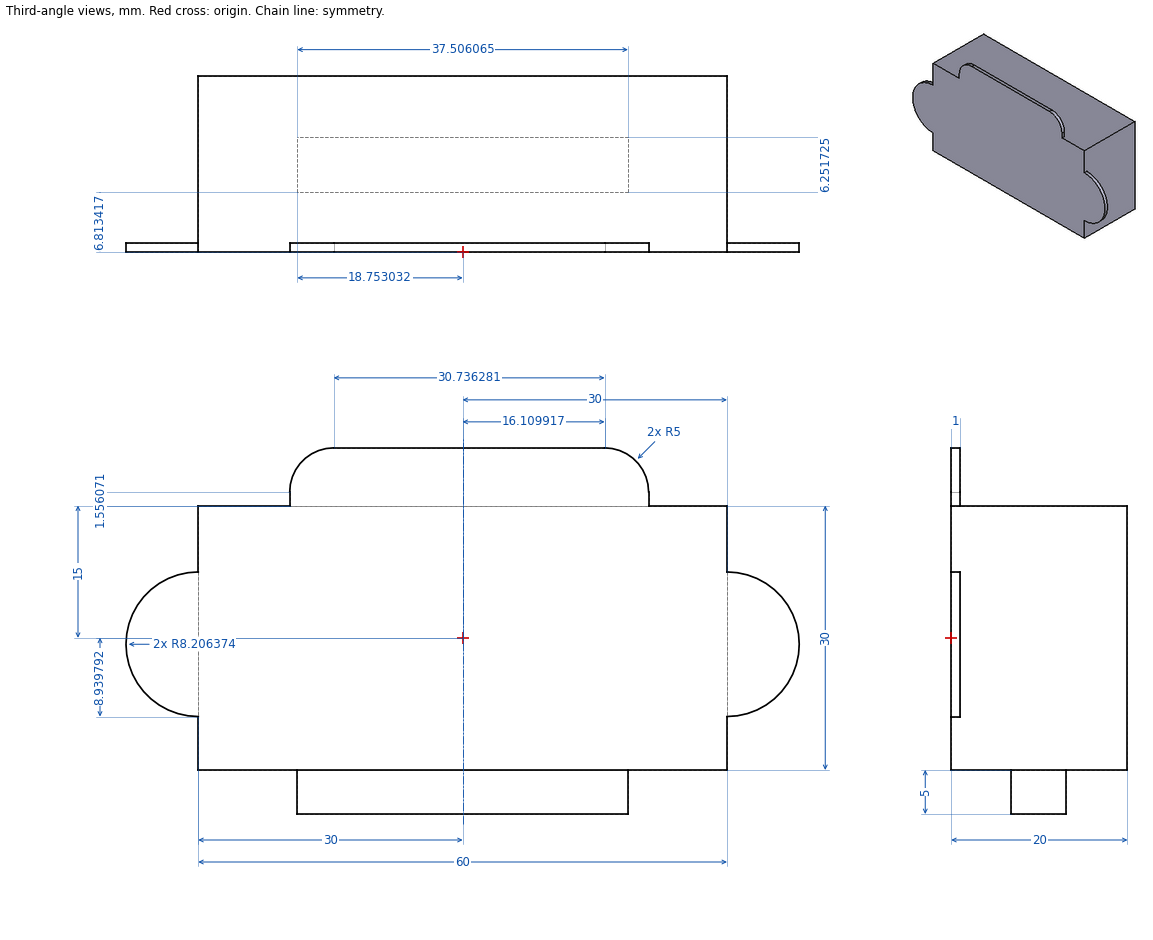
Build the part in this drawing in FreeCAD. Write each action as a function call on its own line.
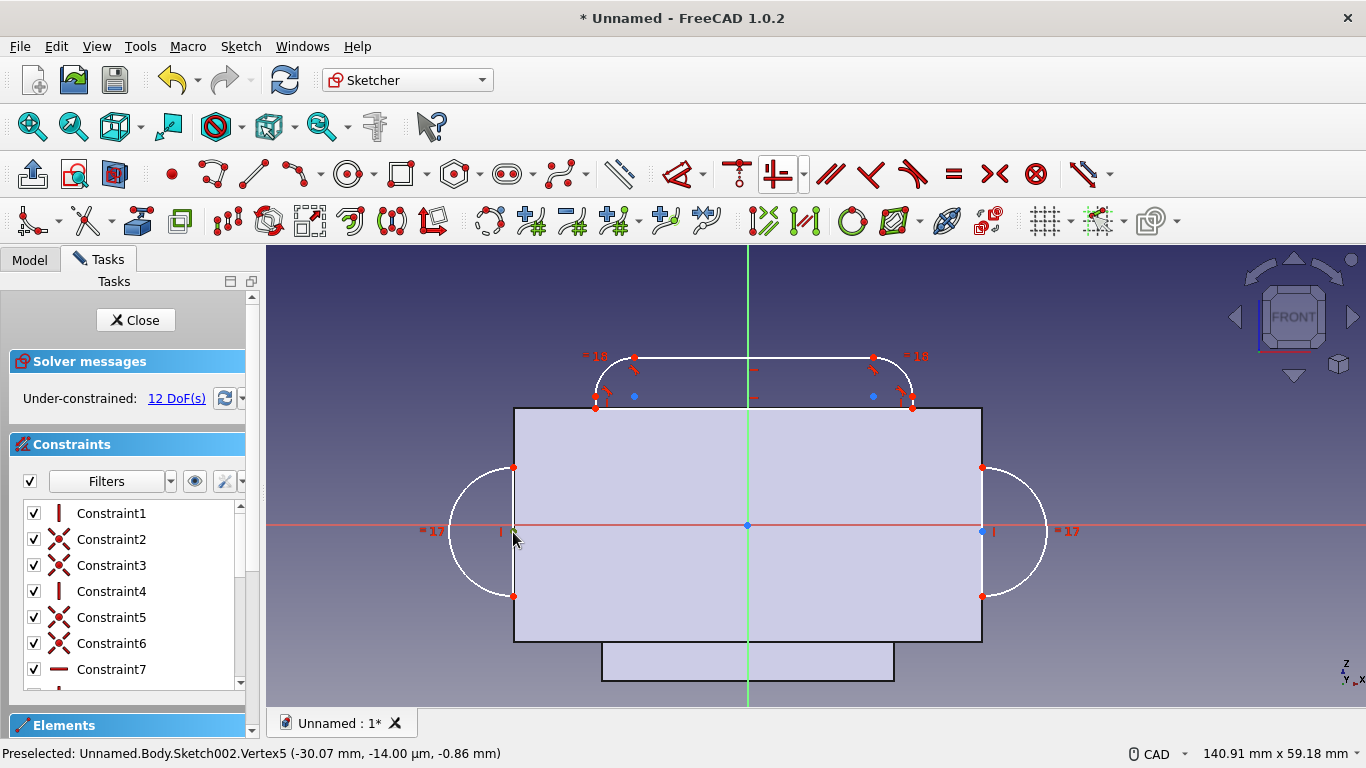
click(983, 532)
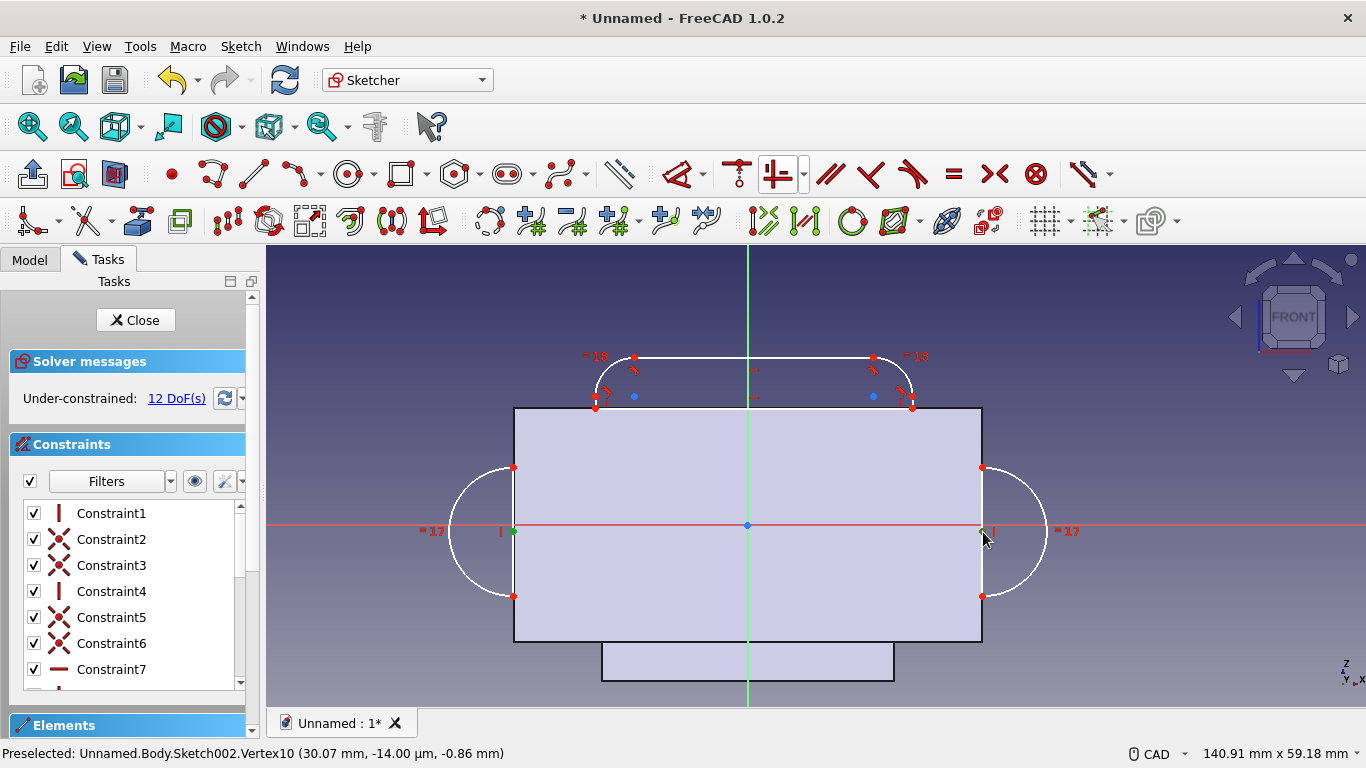
click(748, 650)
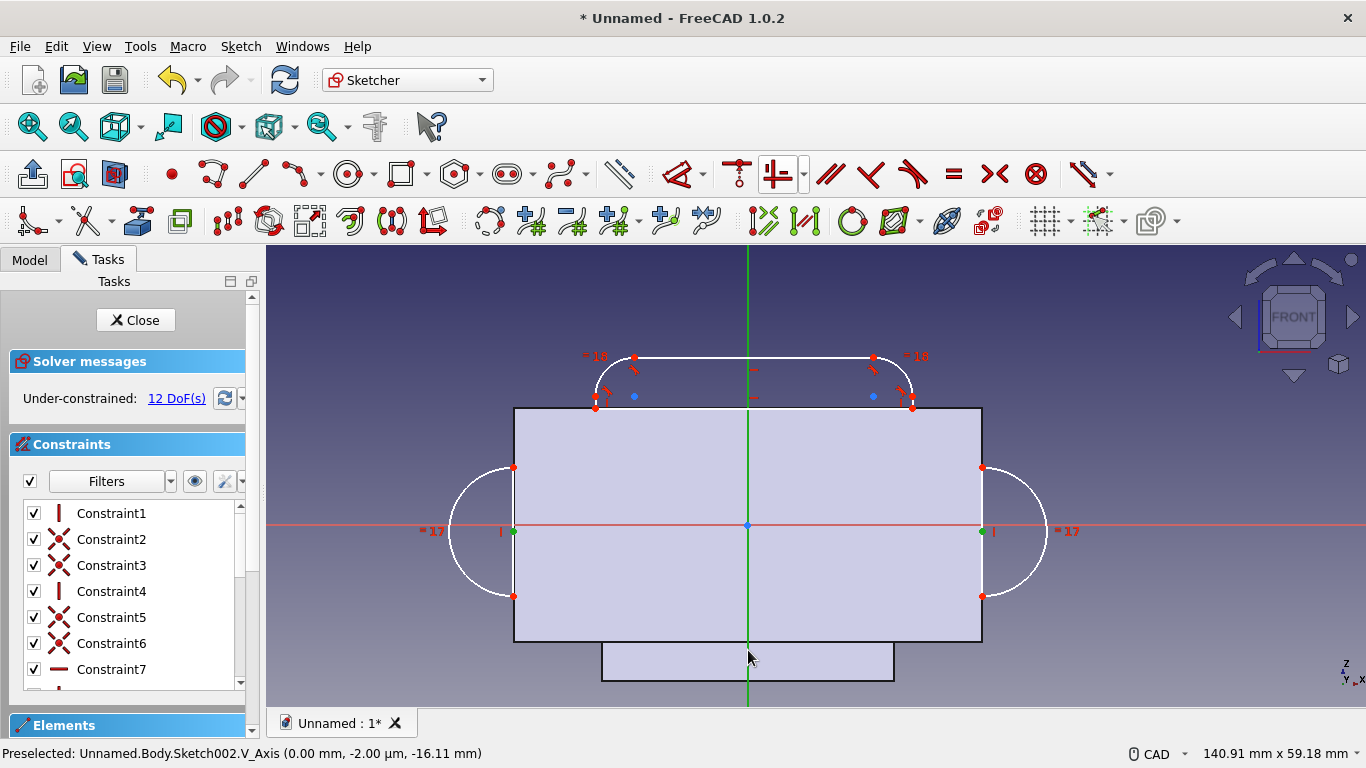
key(s)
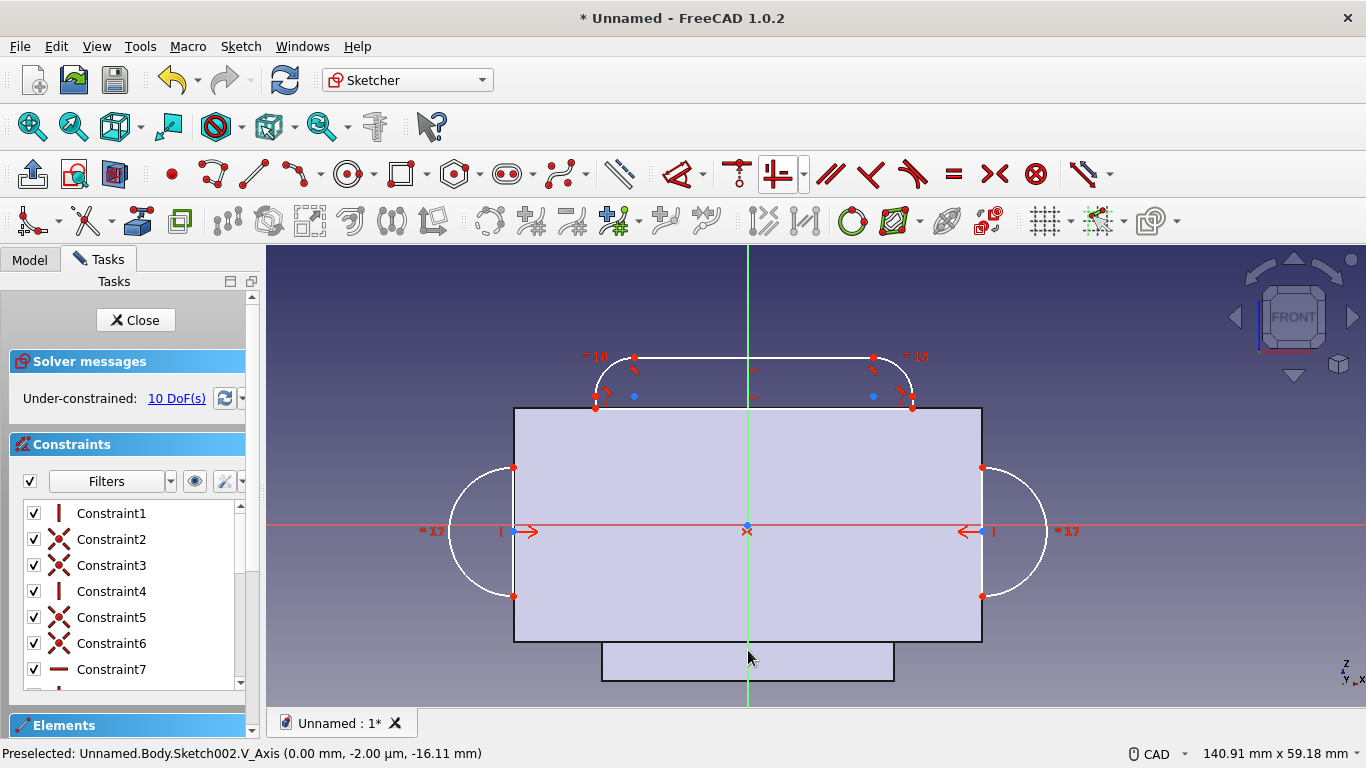
key(d)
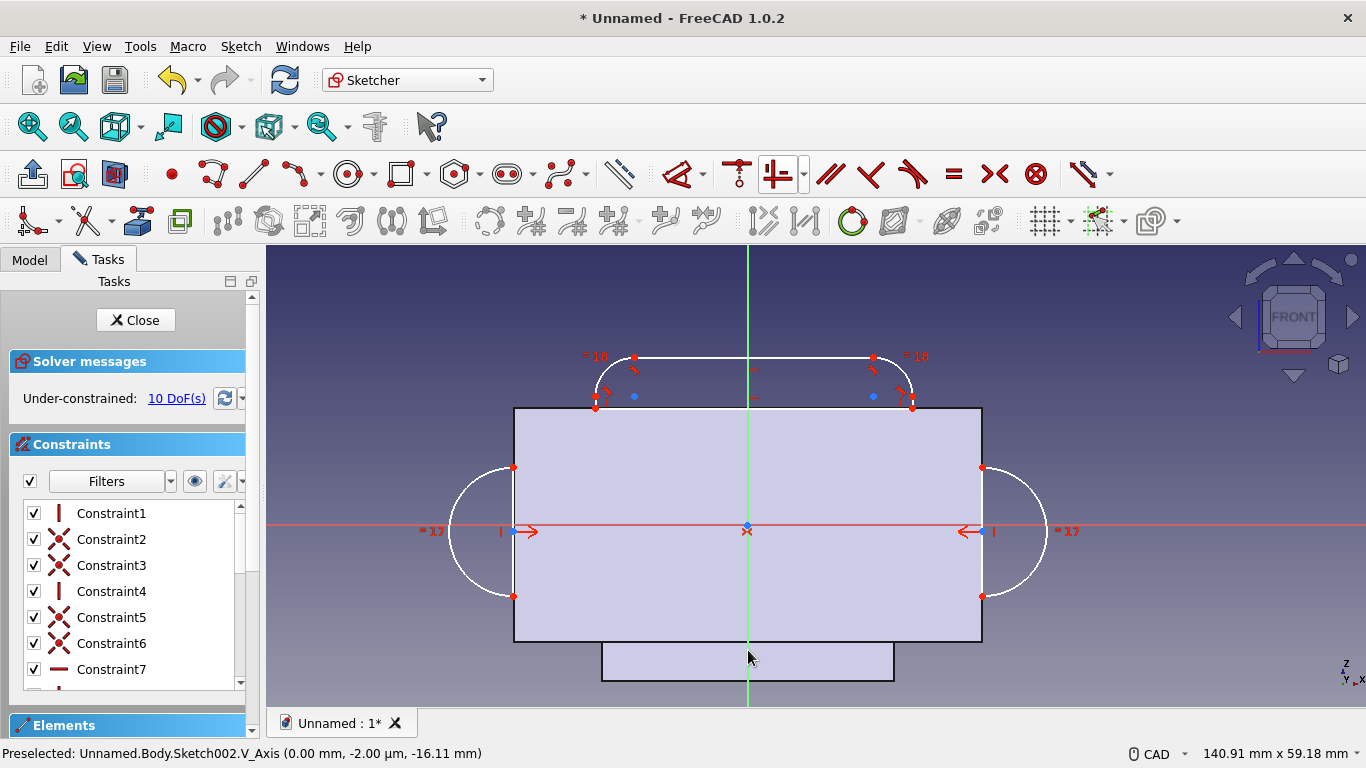
click(461, 494)
click(435, 475)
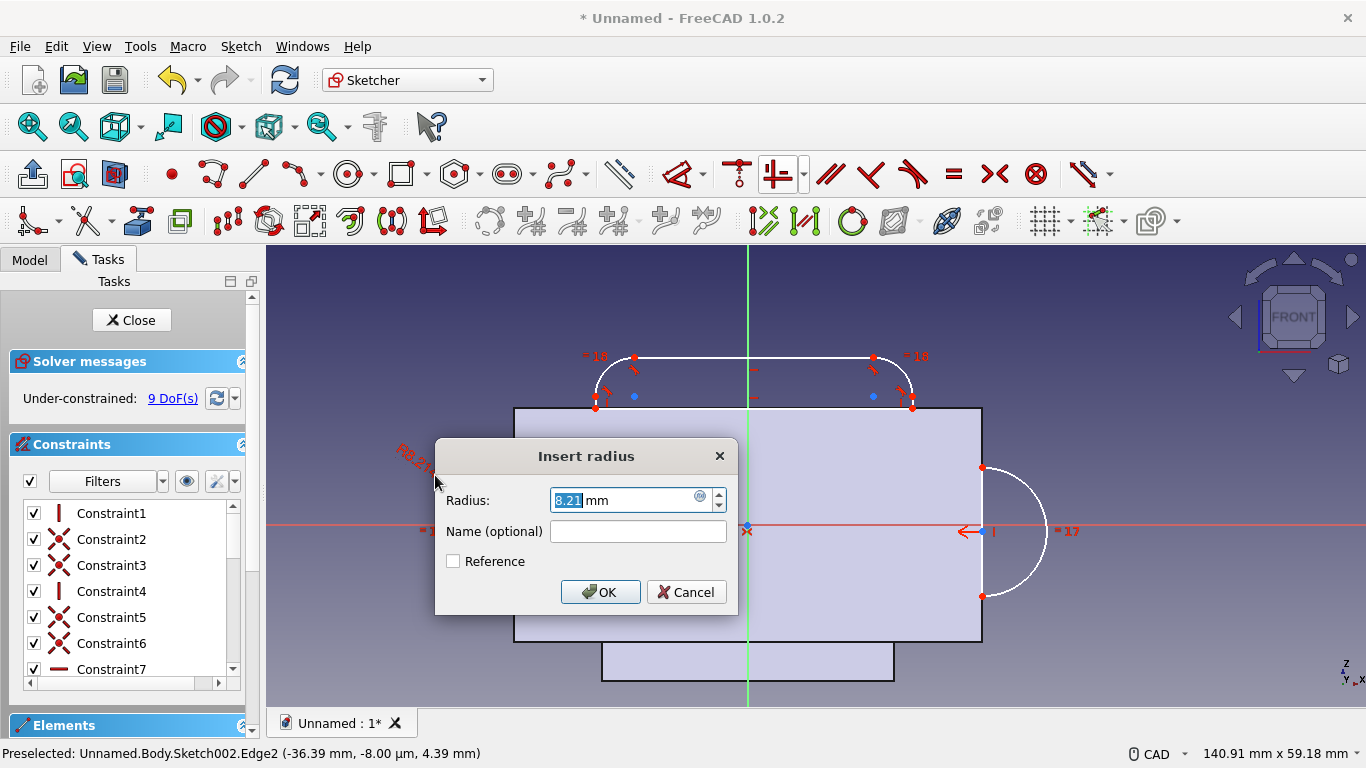
text(8.206374)
key(Return)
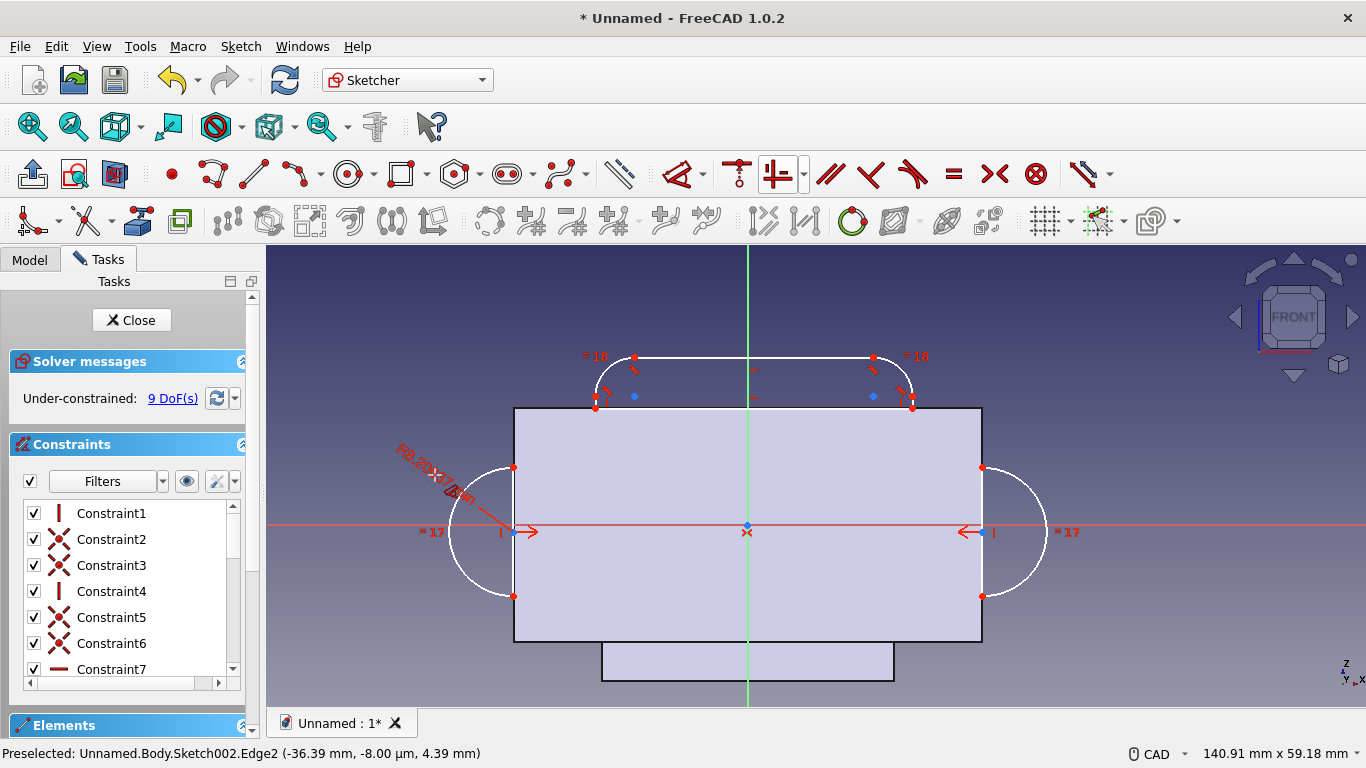
click(617, 362)
click(603, 333)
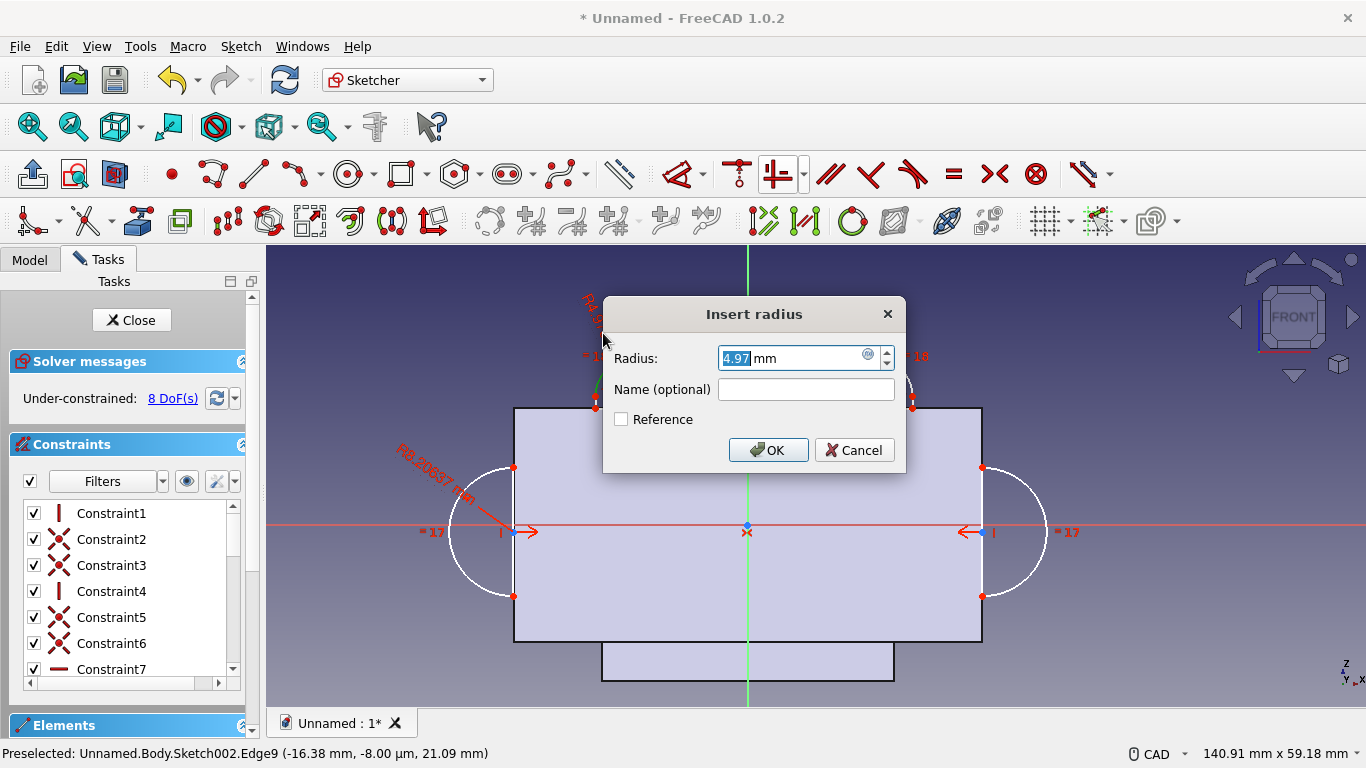
text(5)
key(Return)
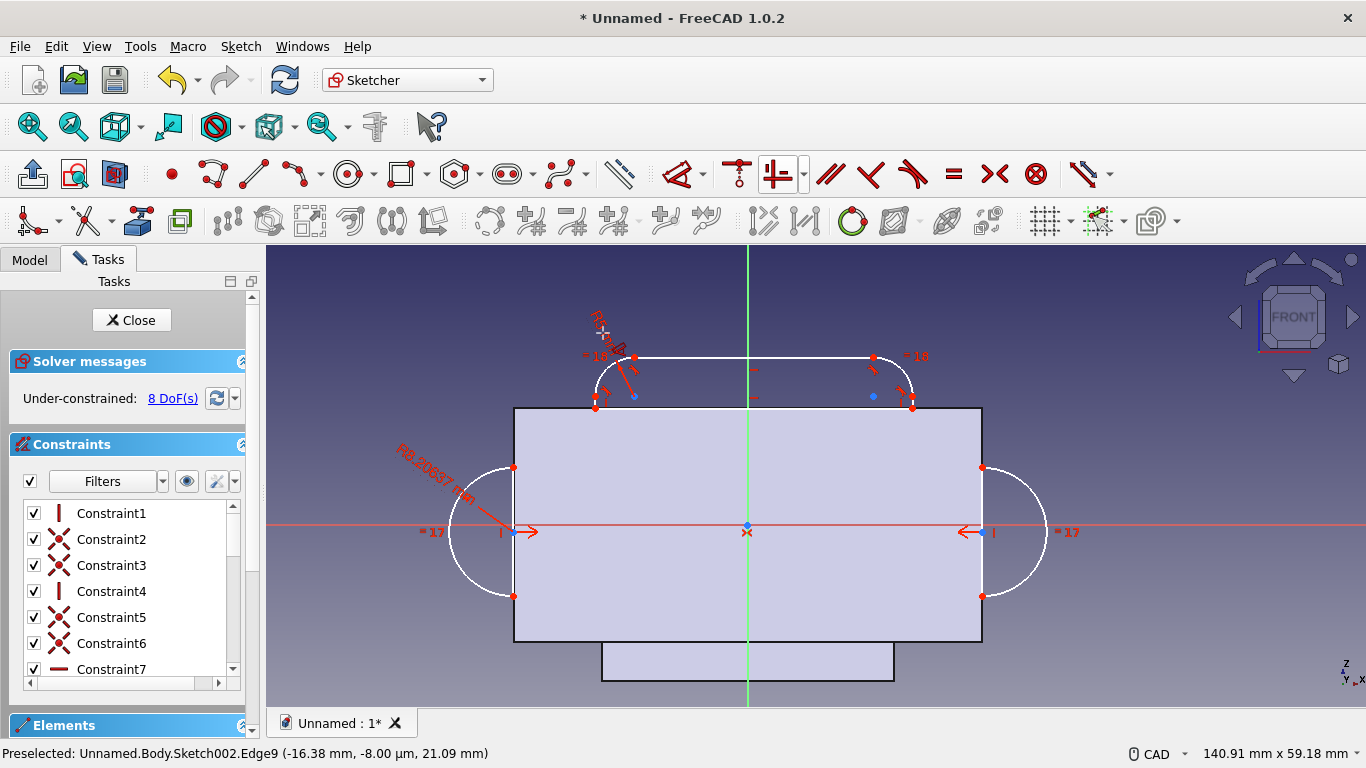
click(513, 596)
click(631, 630)